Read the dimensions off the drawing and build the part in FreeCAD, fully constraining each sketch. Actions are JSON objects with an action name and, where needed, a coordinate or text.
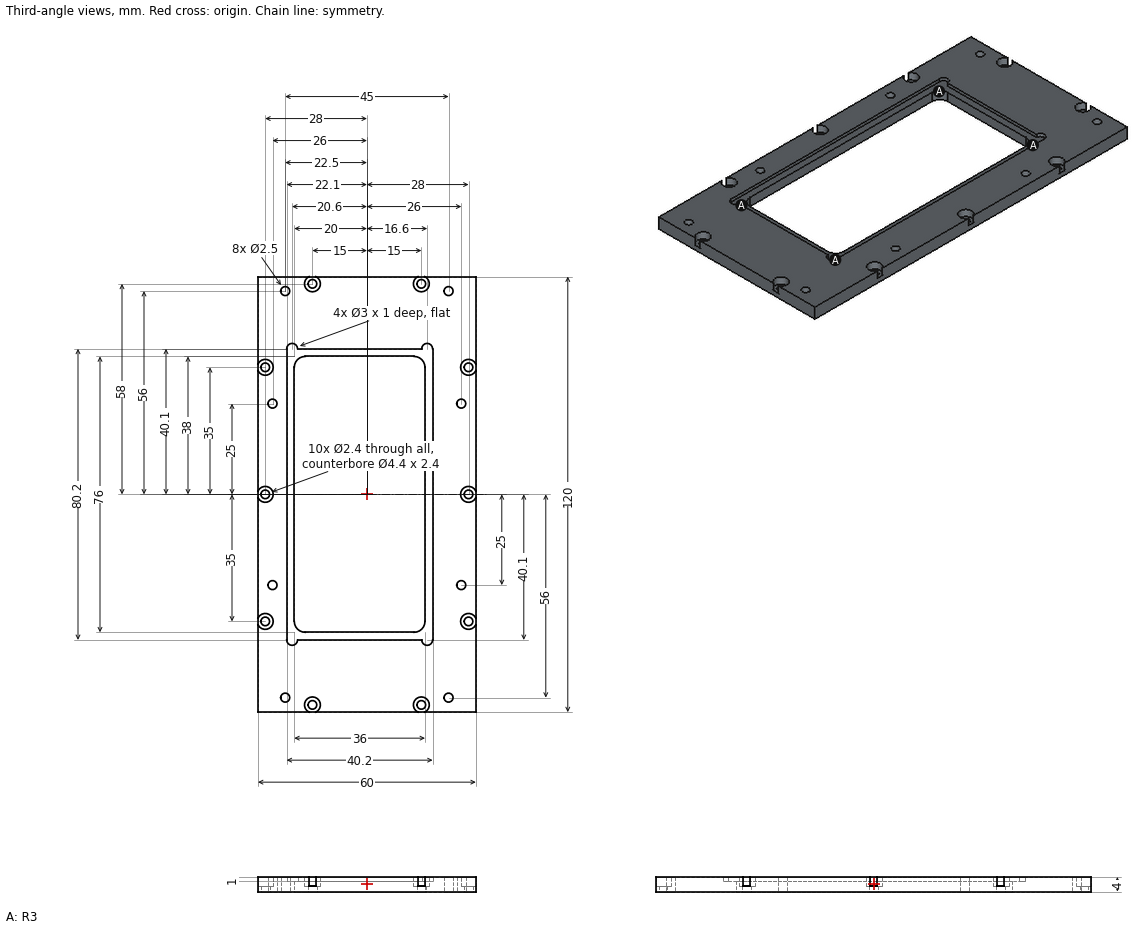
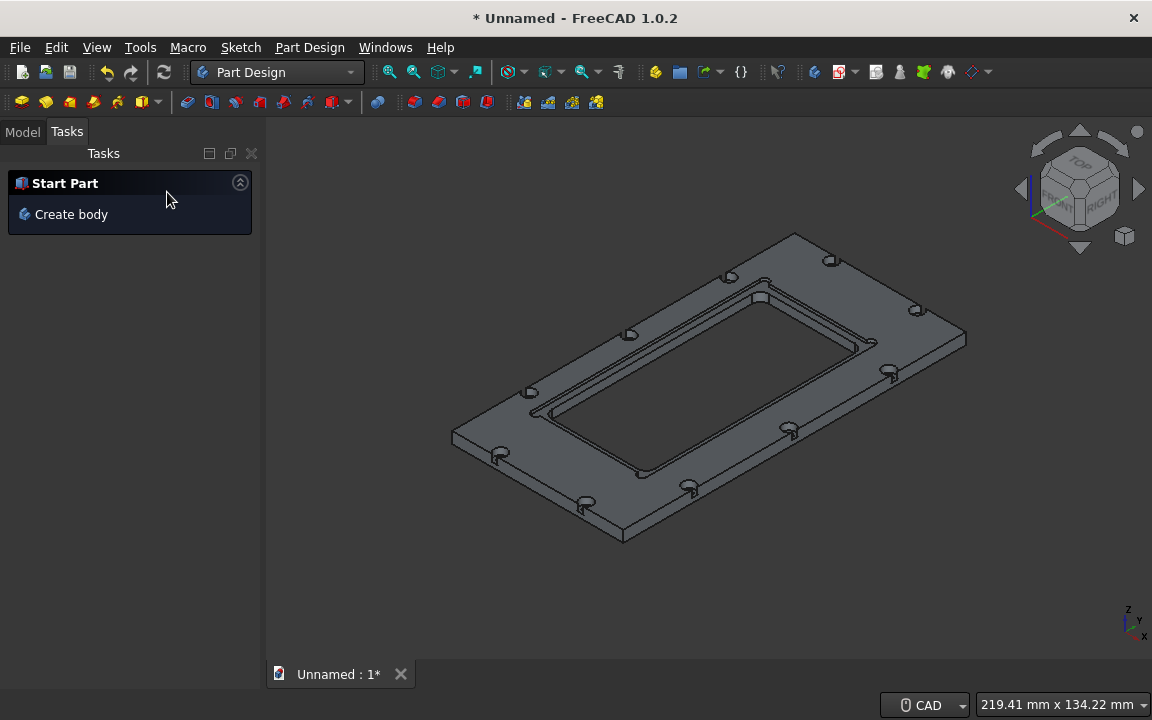
{"action": "left_click", "coordinate": [856, 296]}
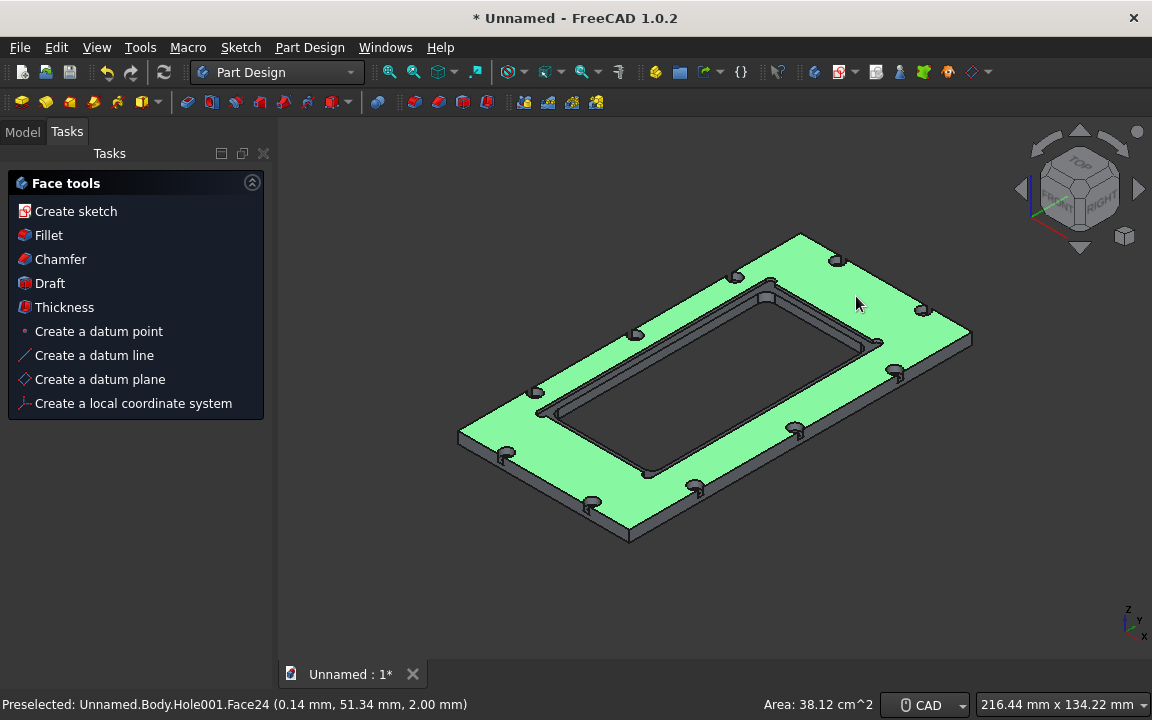
{"action": "left_click", "coordinate": [840, 72]}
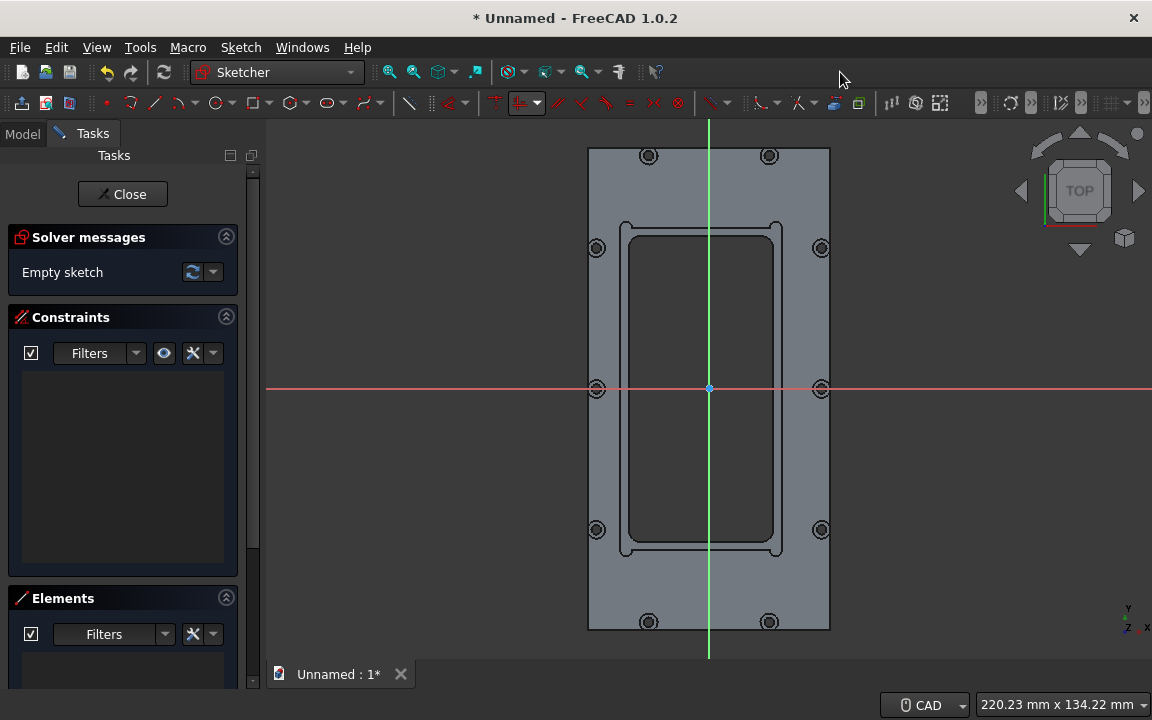
{"action": "scroll", "coordinate": [331, 389], "scroll_direction": "down", "scroll_amount": 1}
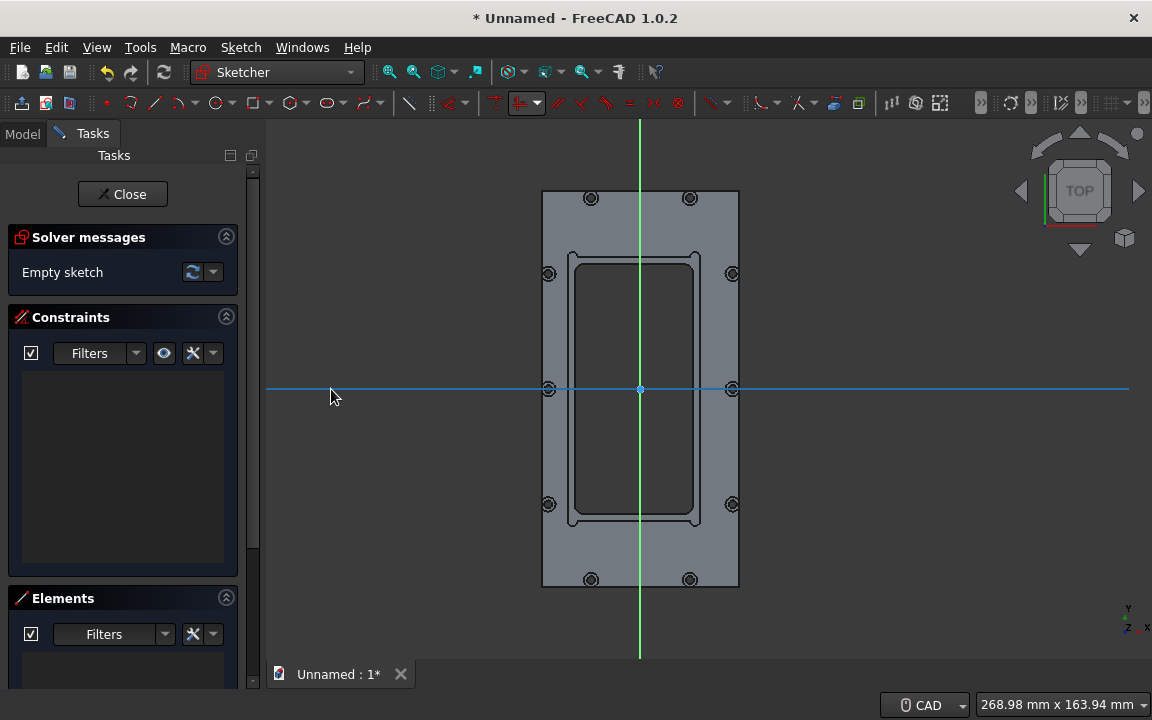
{"action": "key", "text": "g c"}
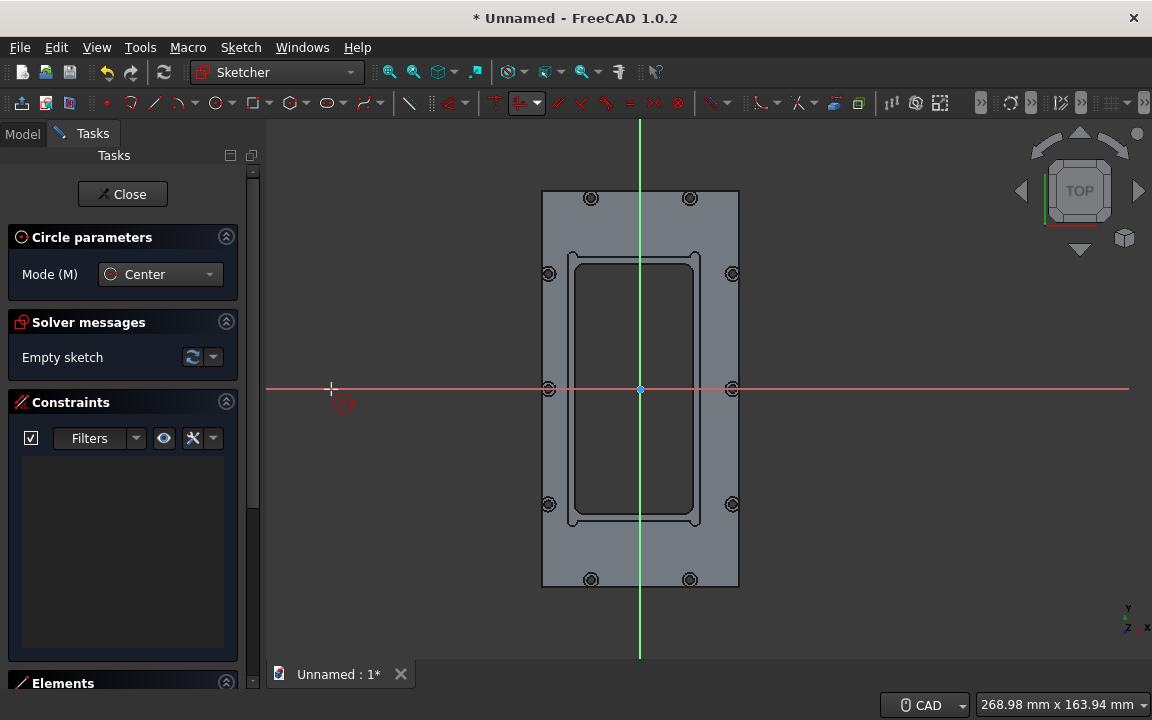
{"action": "scroll", "coordinate": [566, 205], "scroll_direction": "up", "scroll_amount": 9}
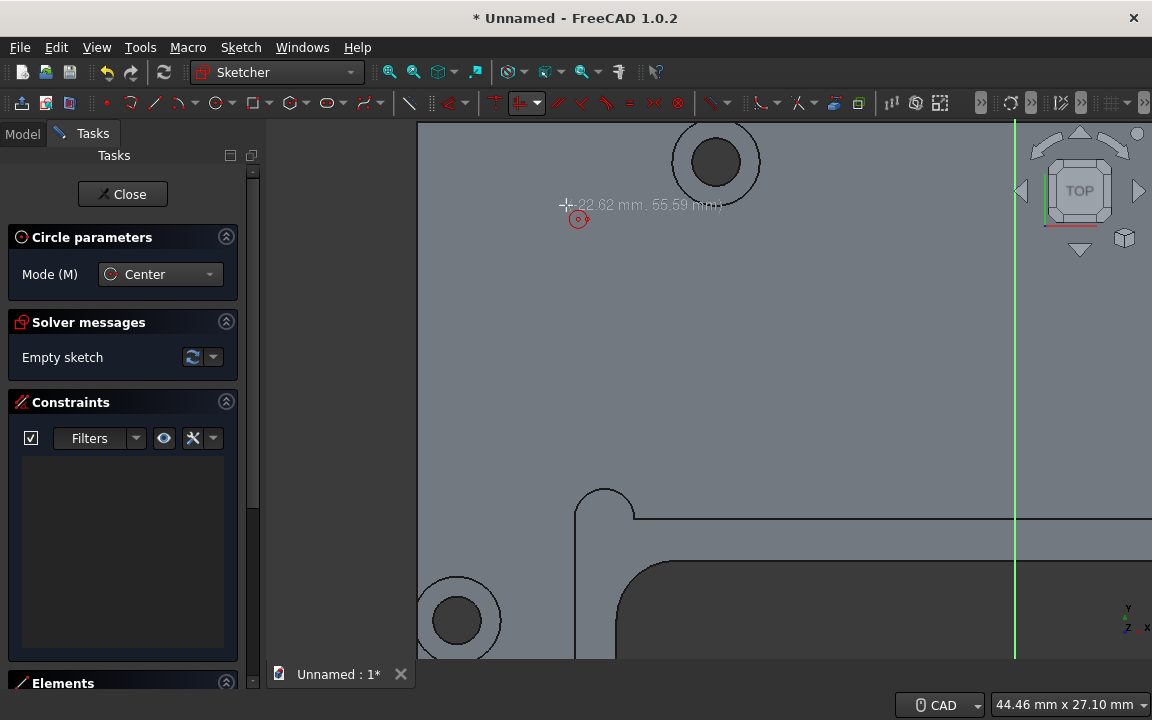
{"action": "scroll", "coordinate": [566, 205], "scroll_direction": "down", "scroll_amount": 9}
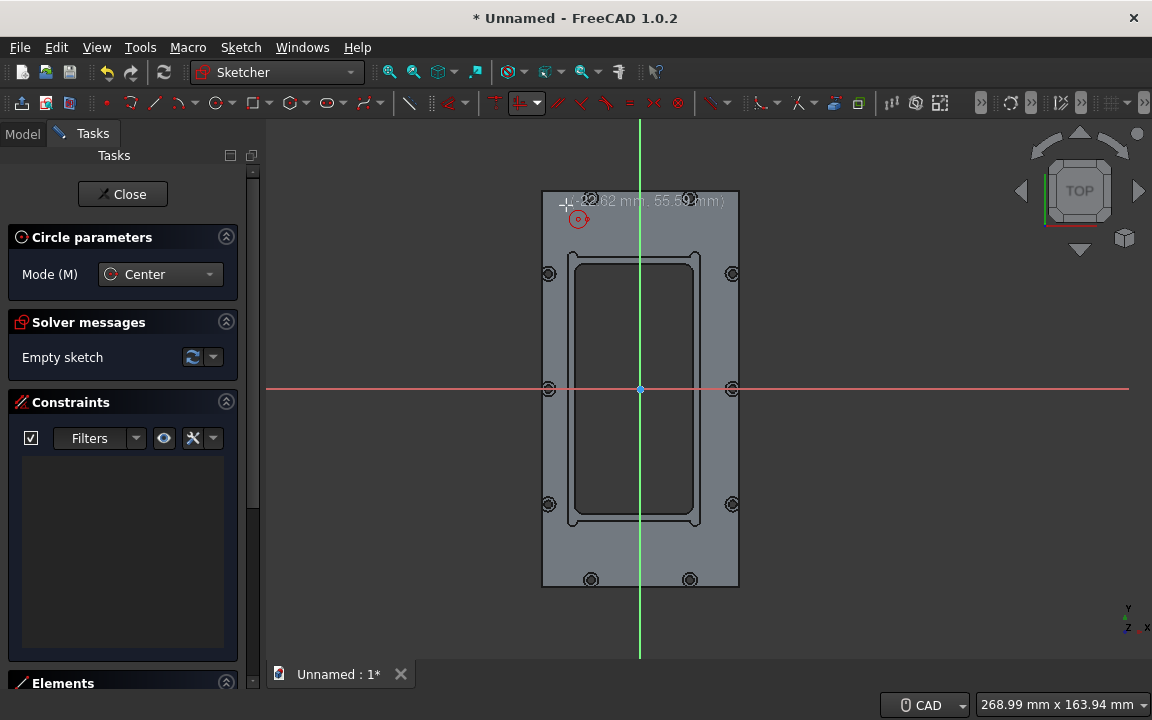
{"action": "left_click", "coordinate": [566, 205]}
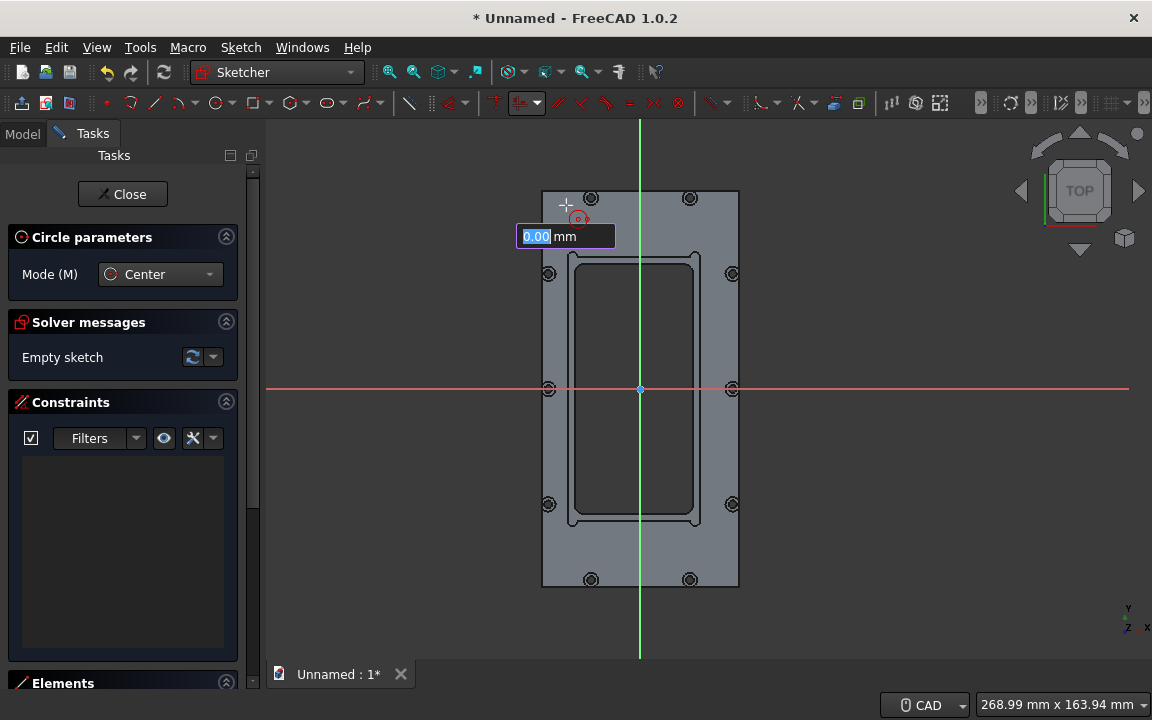
{"action": "scroll", "coordinate": [569, 202], "scroll_direction": "up", "scroll_amount": 7}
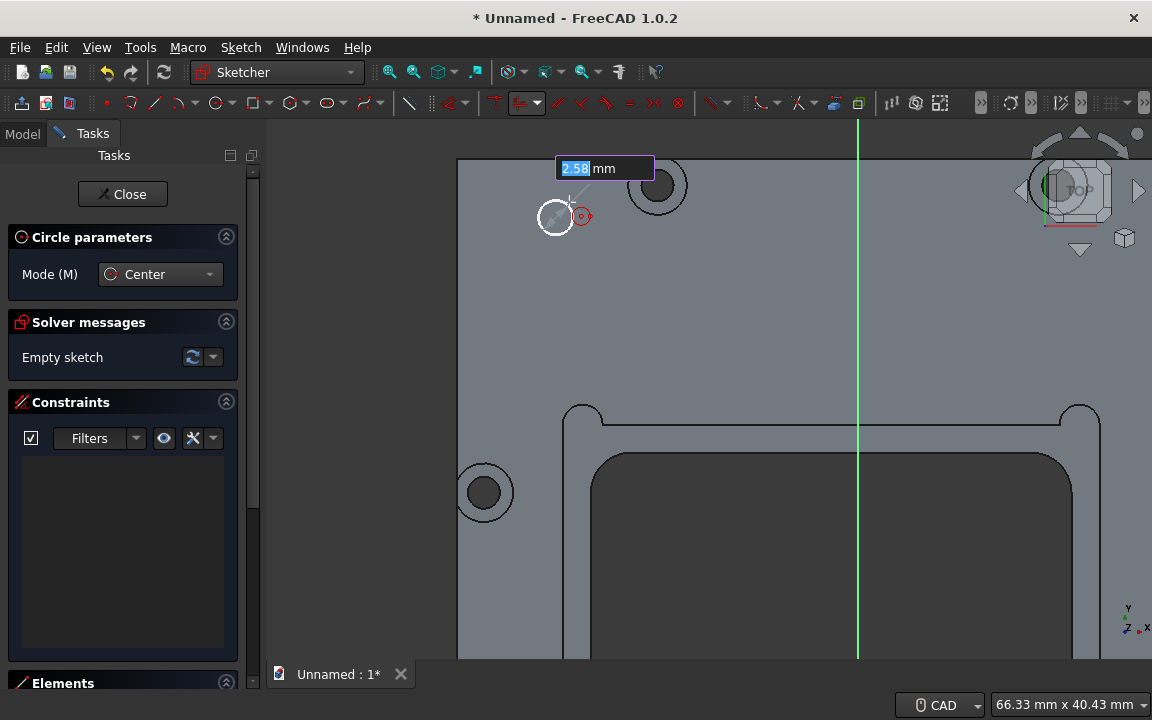
{"action": "left_click", "coordinate": [569, 200]}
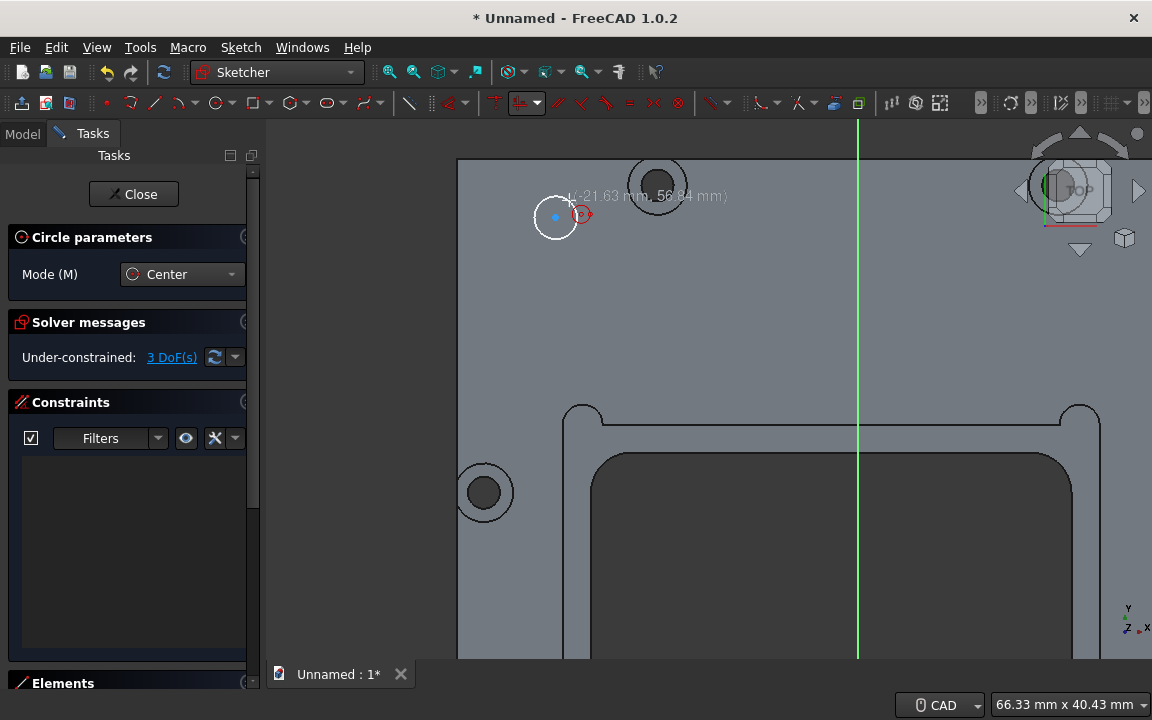
{"action": "scroll", "coordinate": [569, 202], "scroll_direction": "down", "scroll_amount": 7}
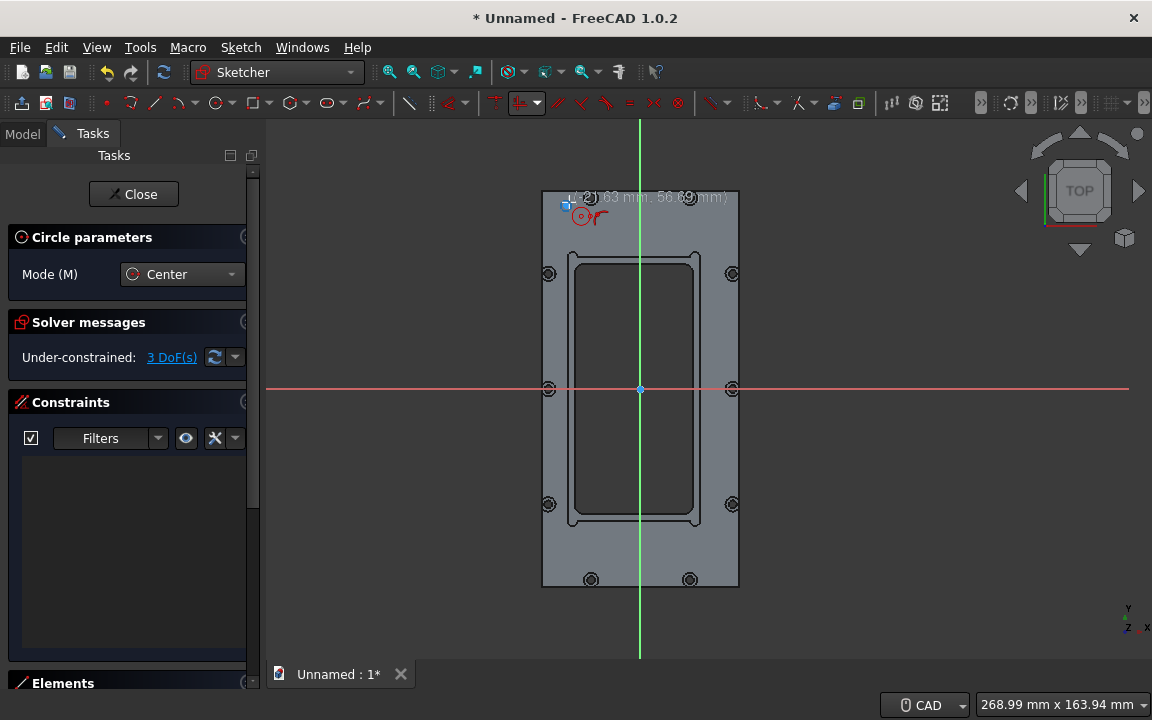
{"action": "scroll", "coordinate": [715, 205], "scroll_direction": "up", "scroll_amount": 9}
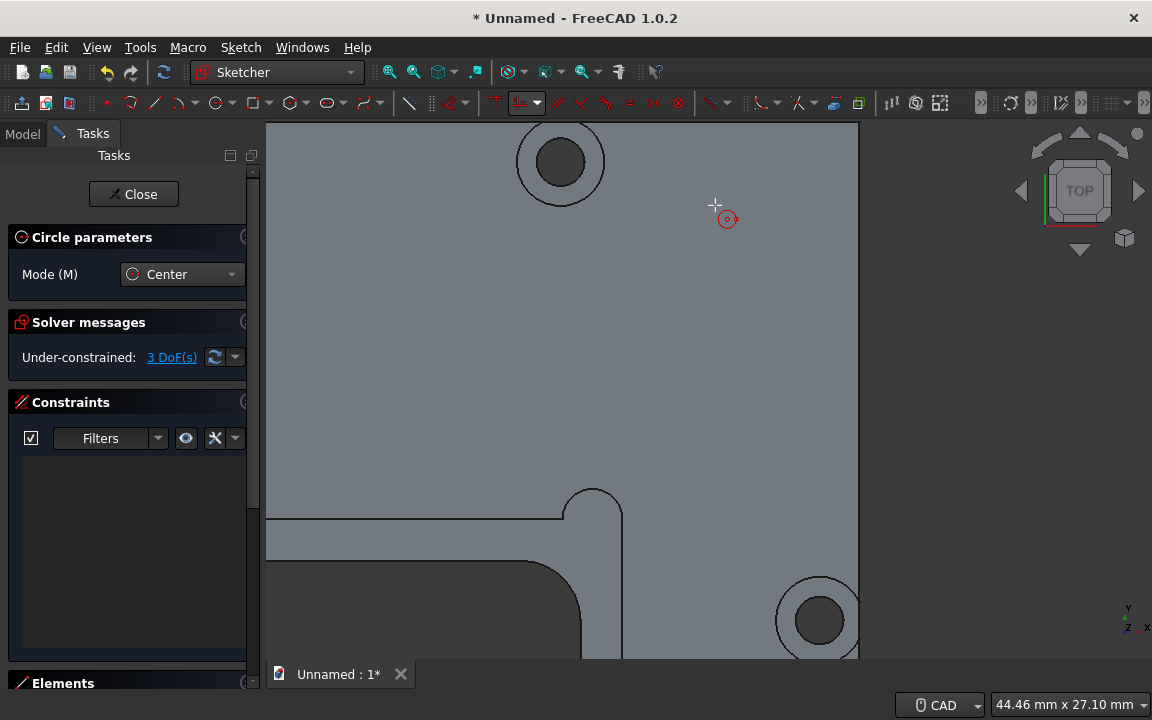
{"action": "scroll", "coordinate": [716, 205], "scroll_direction": "down", "scroll_amount": 9}